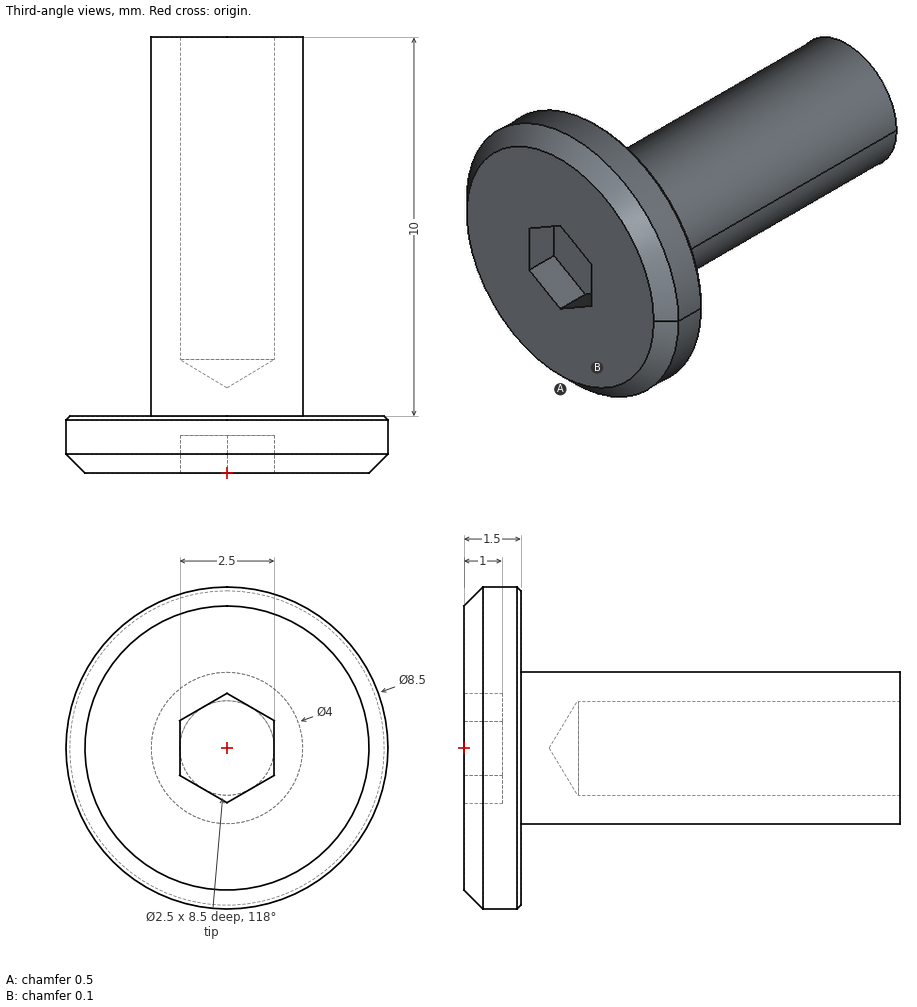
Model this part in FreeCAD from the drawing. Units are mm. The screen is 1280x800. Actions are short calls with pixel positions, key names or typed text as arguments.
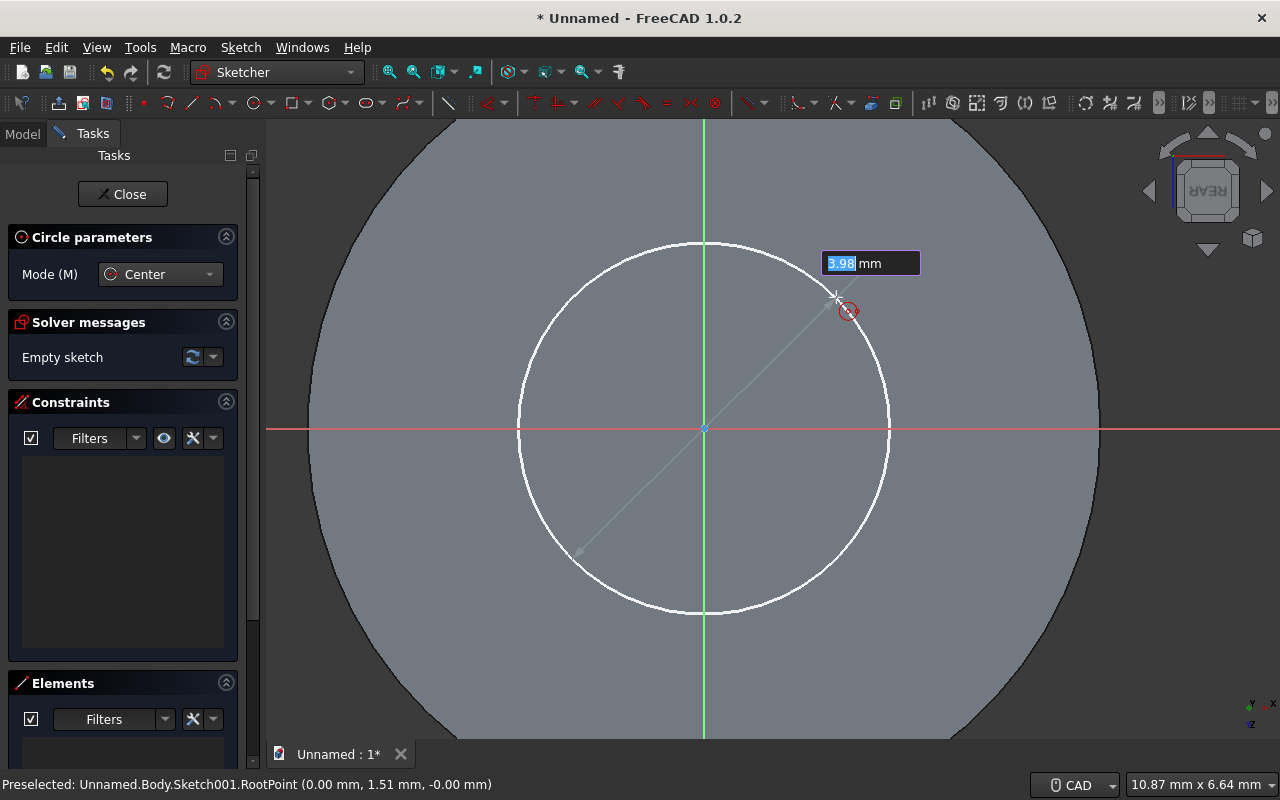
text(4)
key(Return)
key(Escape)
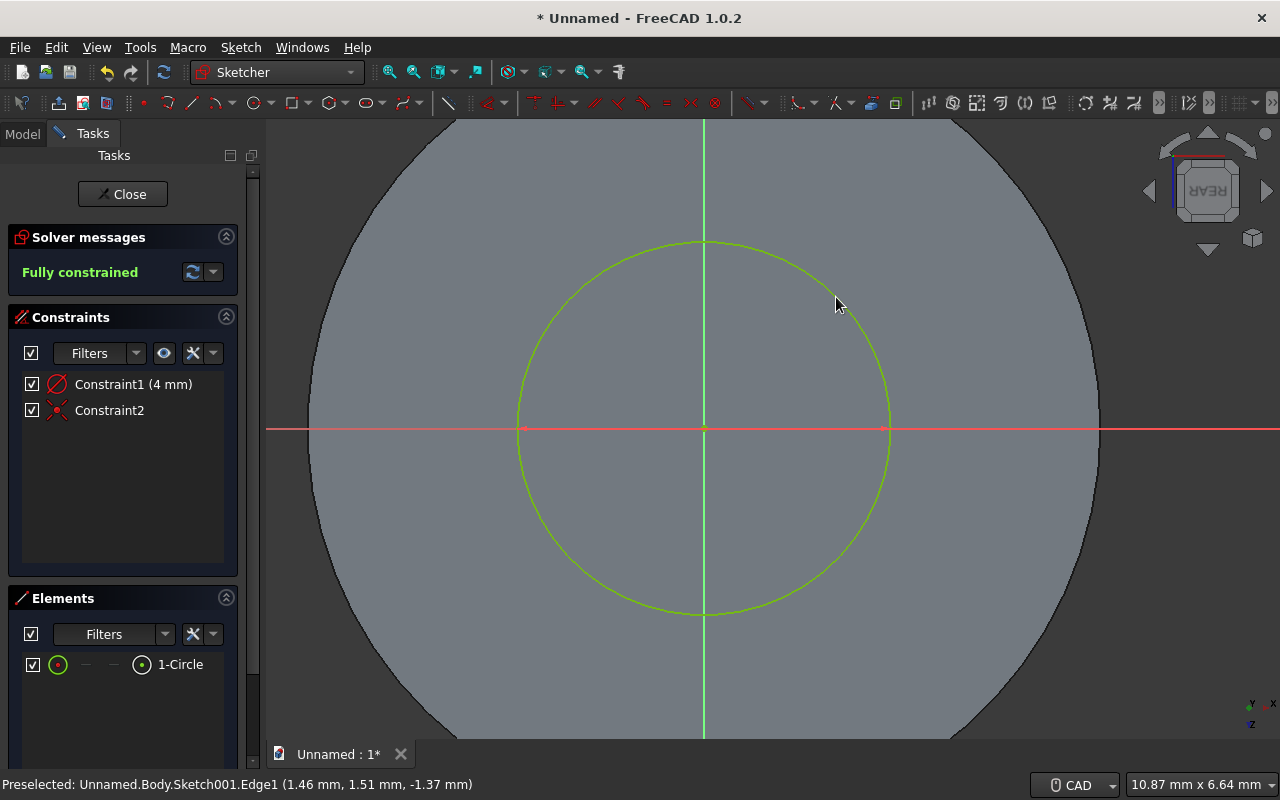
click(123, 194)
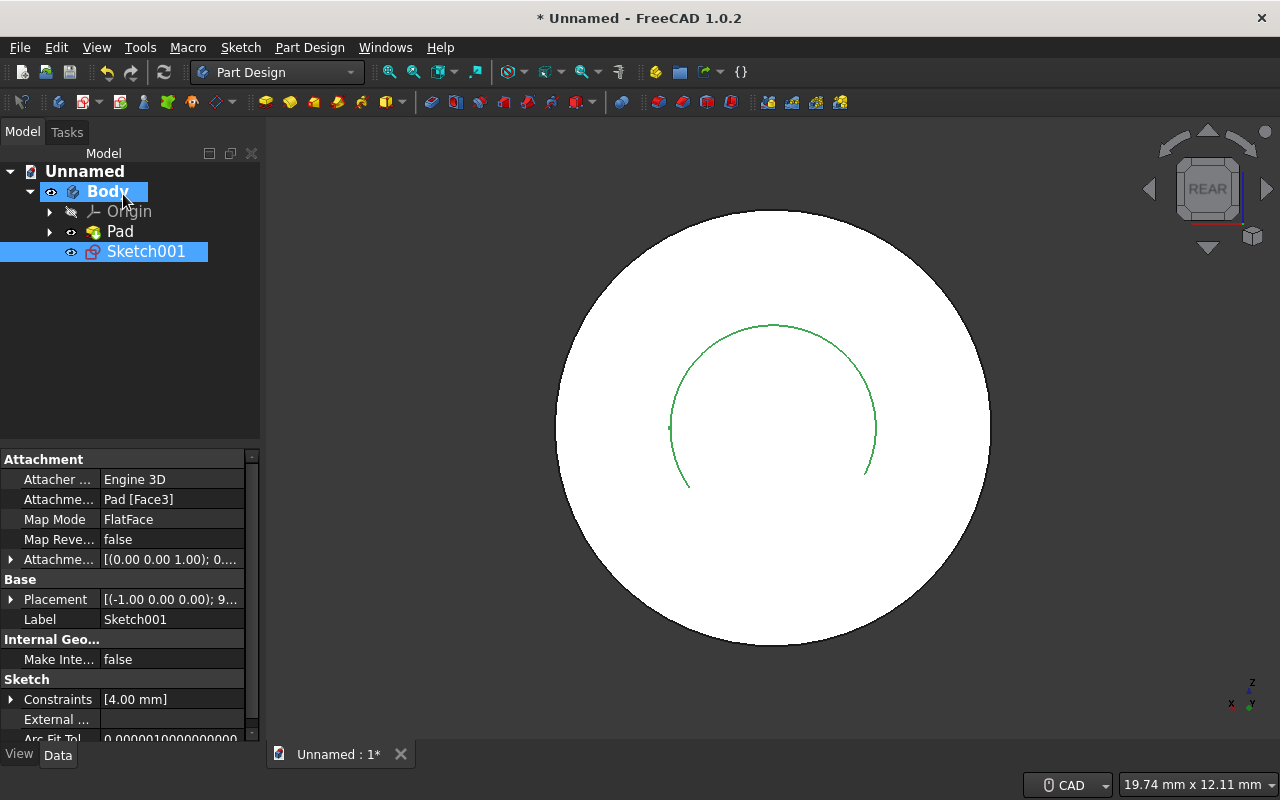
click(266, 102)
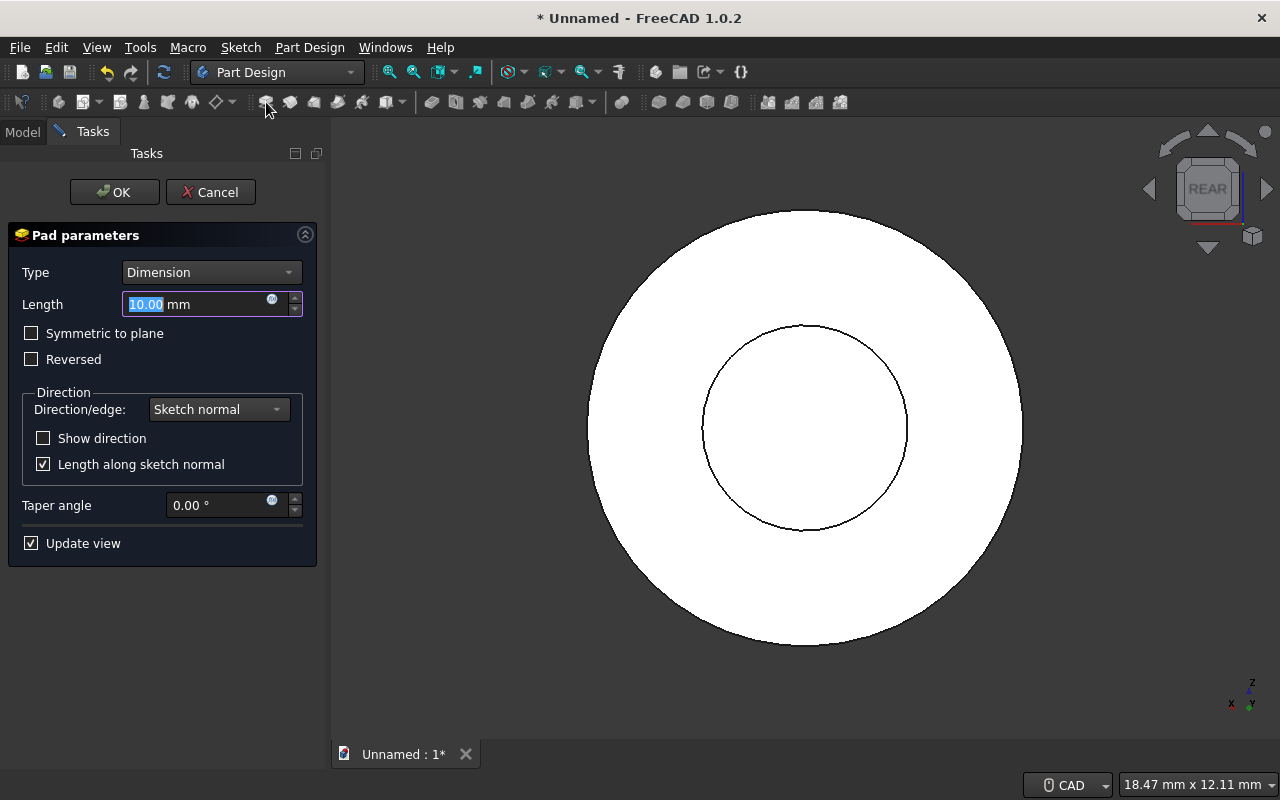
text(10)
key(Tab)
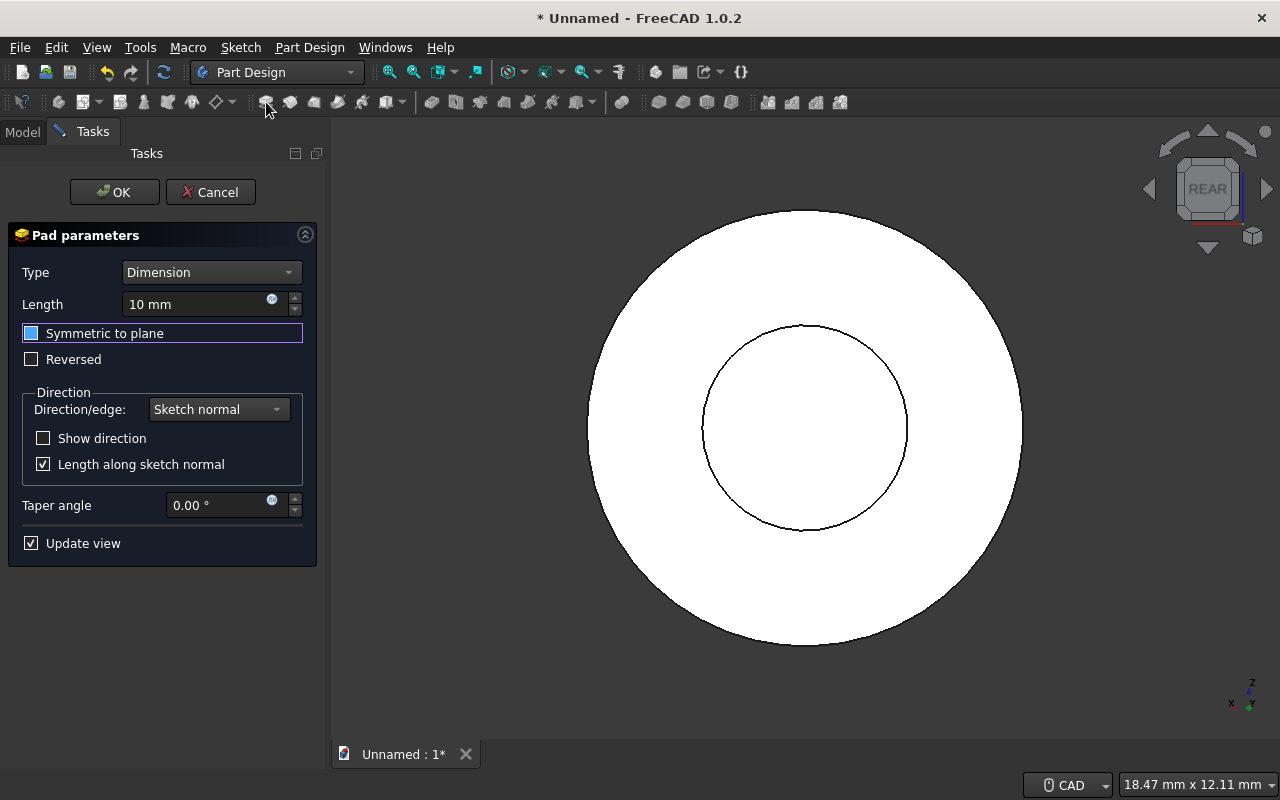
click(115, 192)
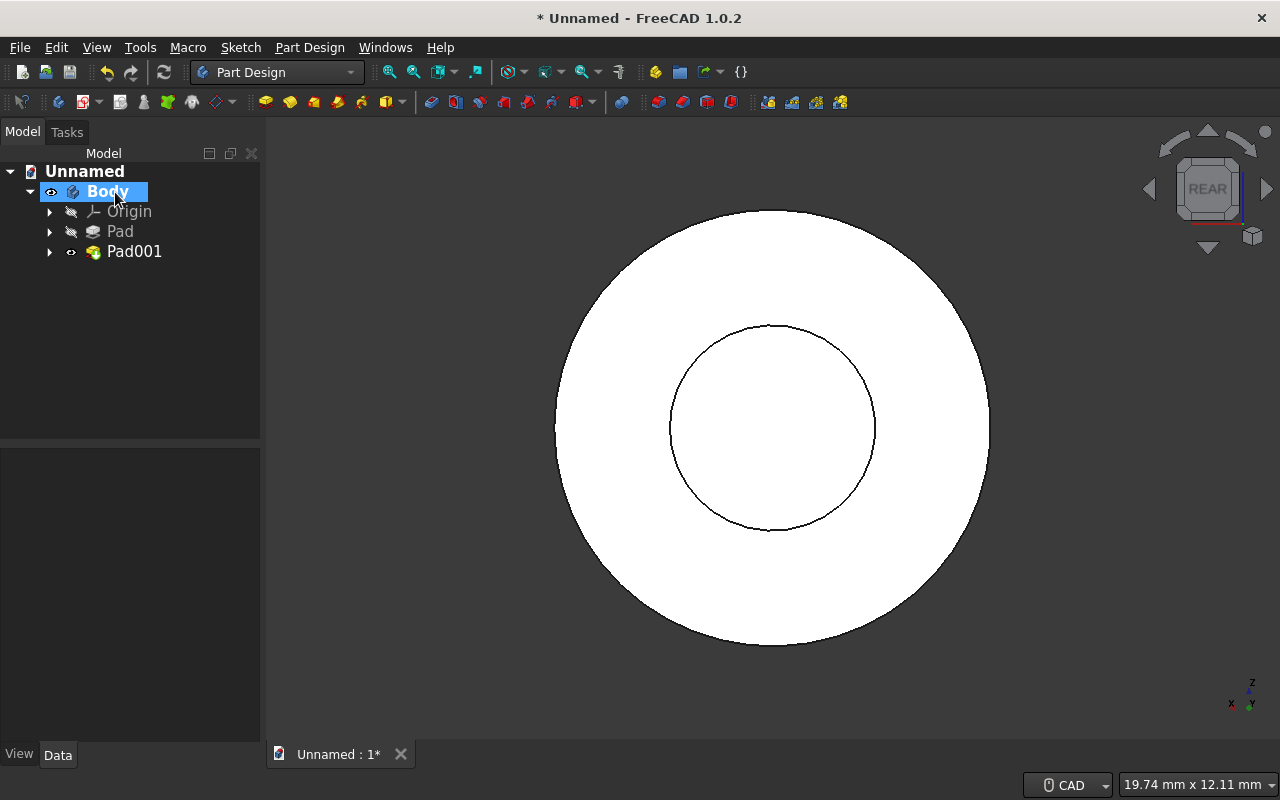
click(773, 427)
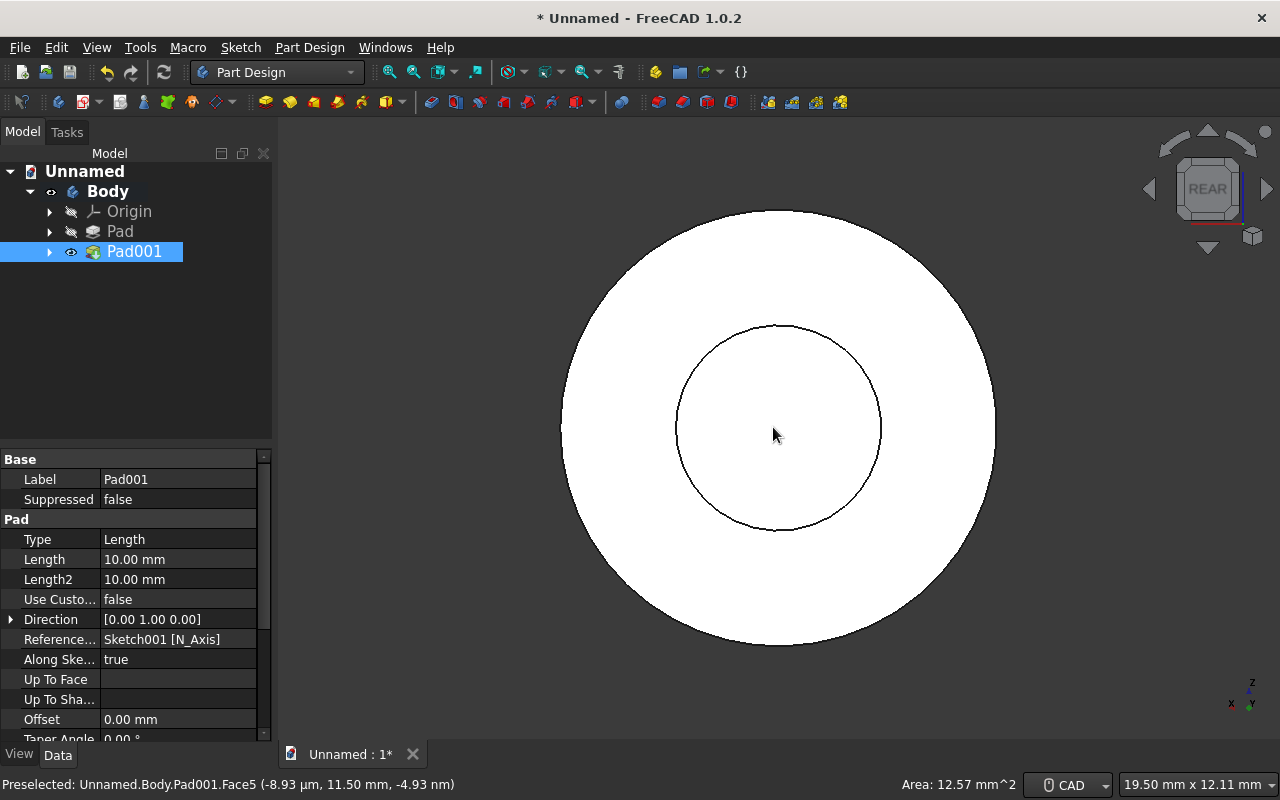
click(84, 102)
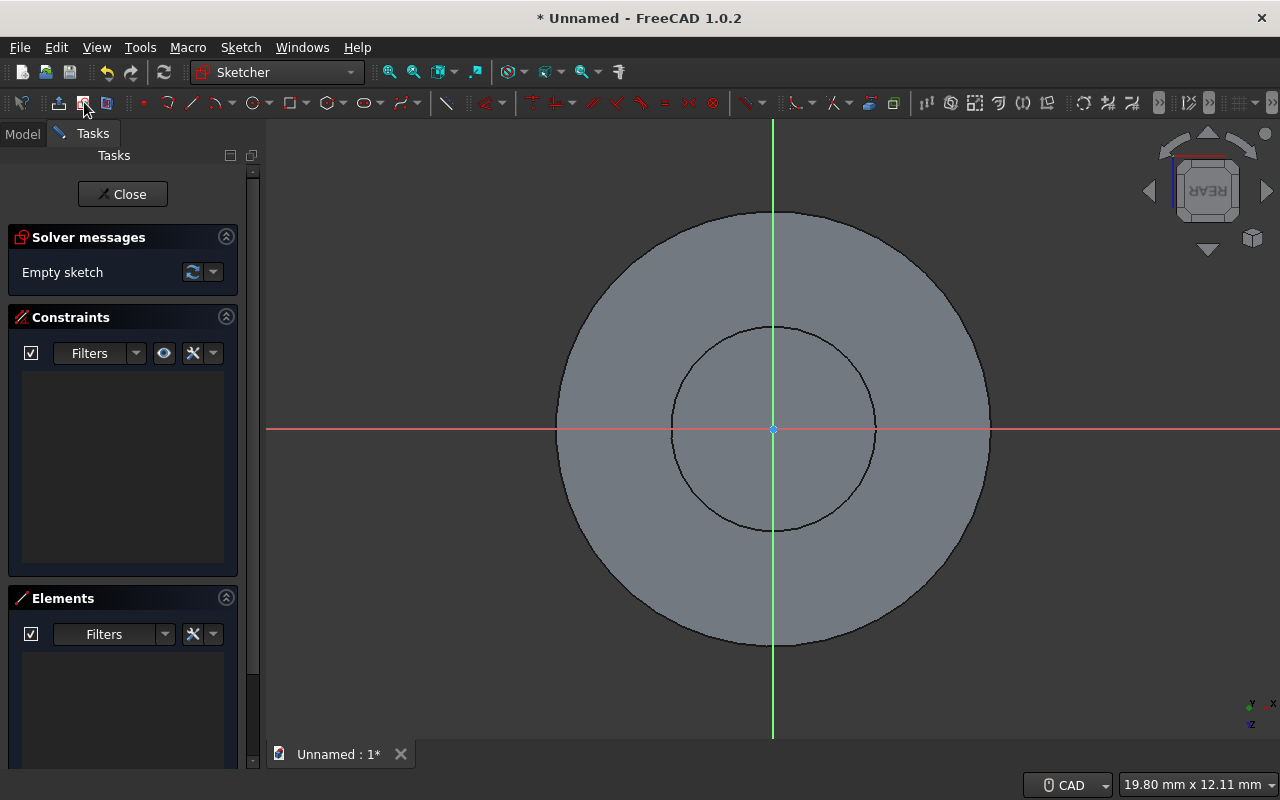
scroll(803, 429, up, 6)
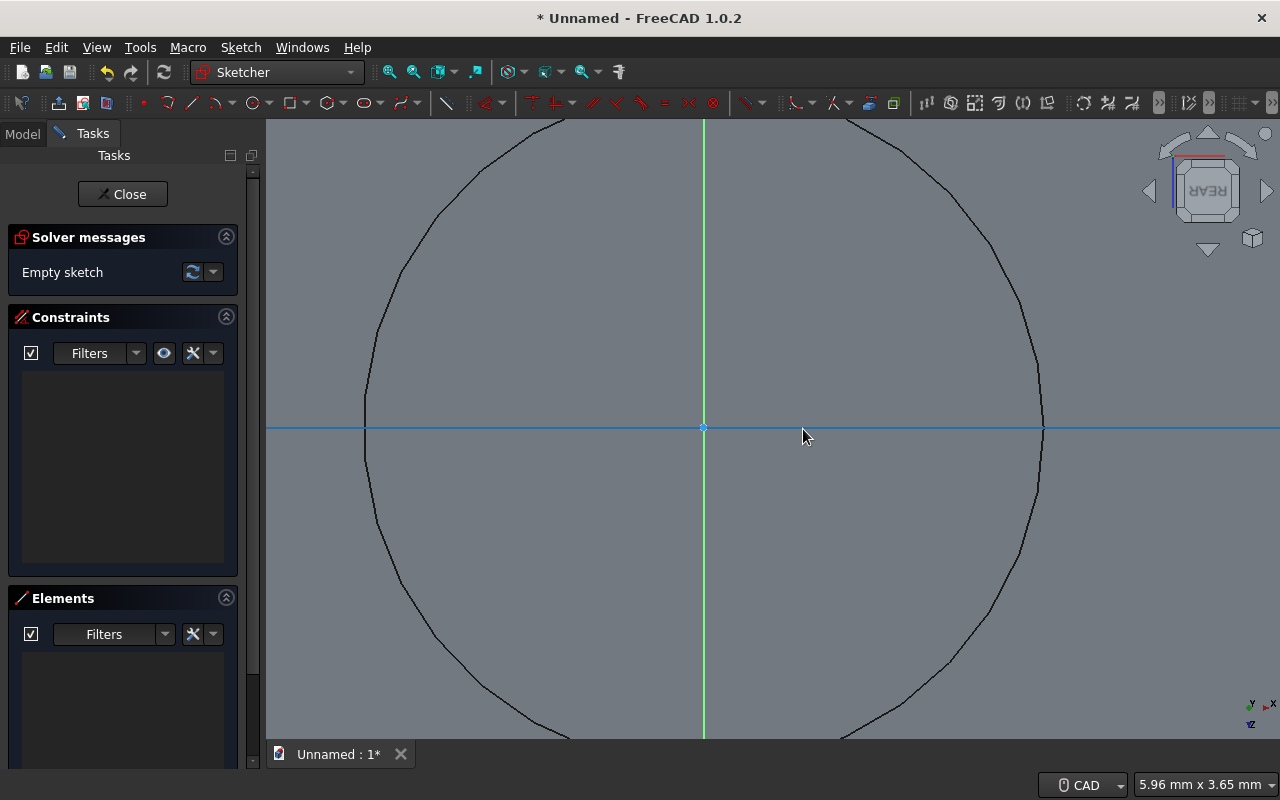
key(g)
key(c)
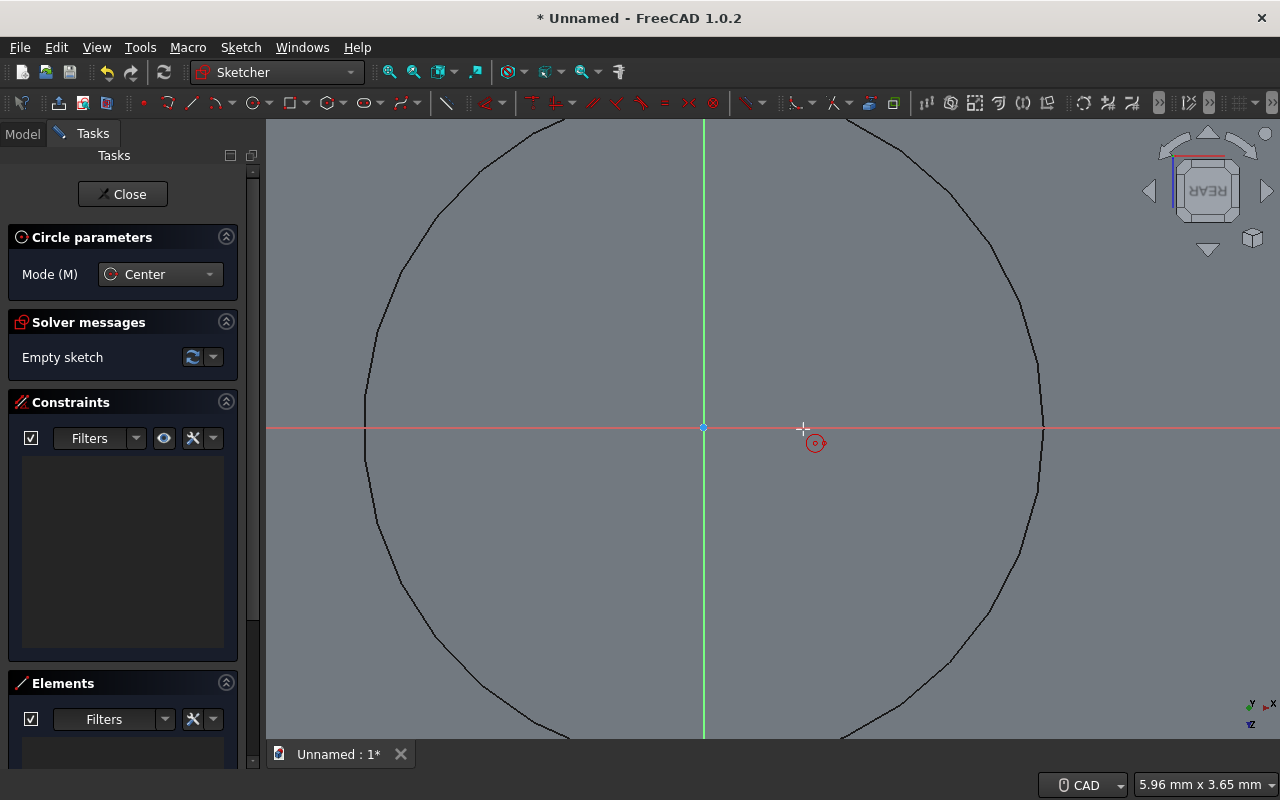
click(704, 428)
move(854, 278)